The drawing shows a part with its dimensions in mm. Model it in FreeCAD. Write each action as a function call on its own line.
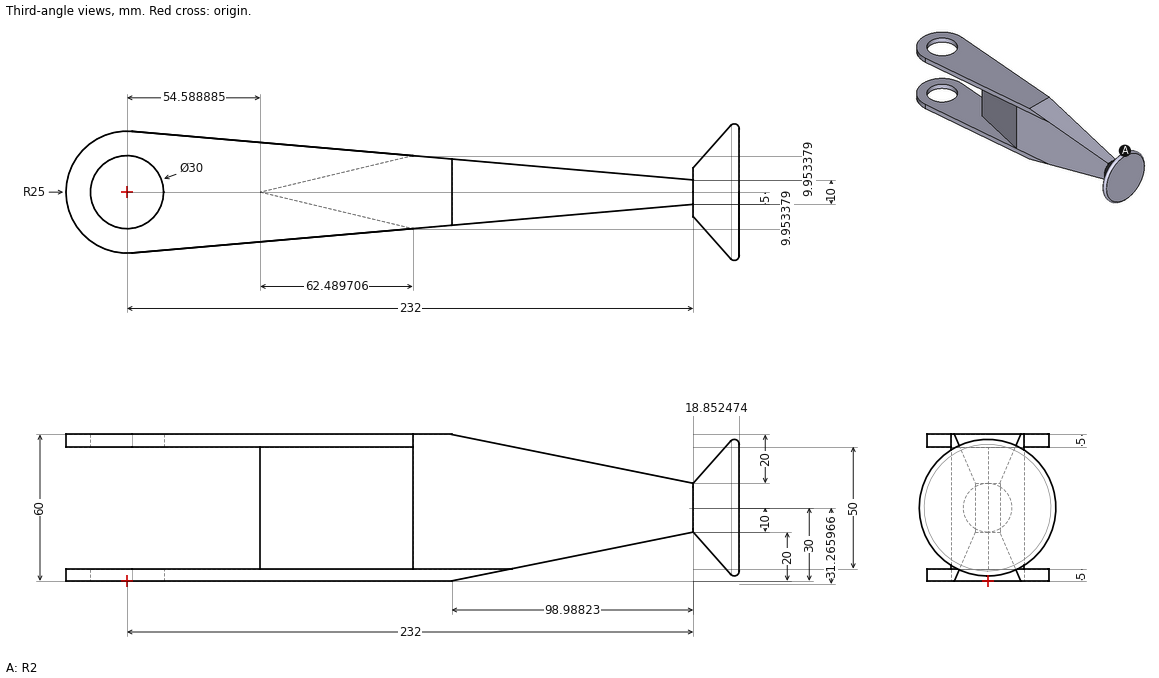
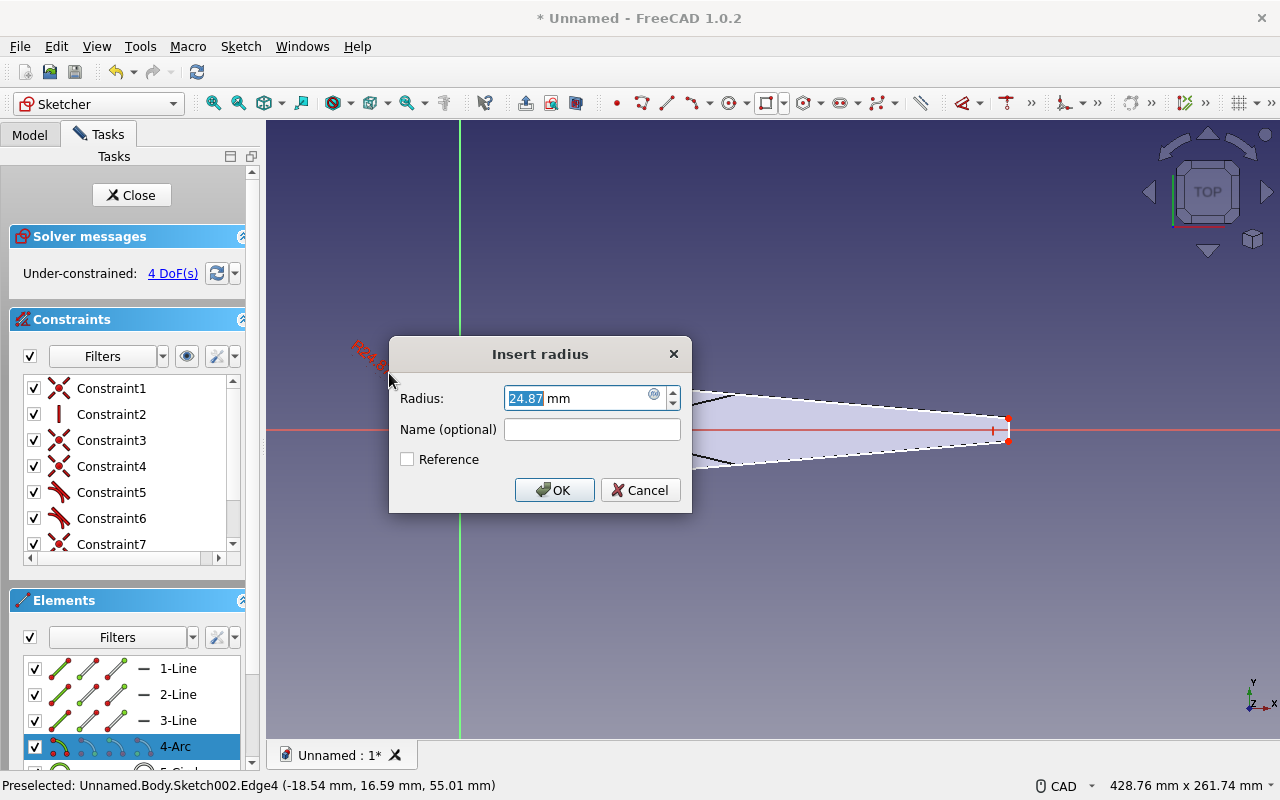
text(25)
key(Return)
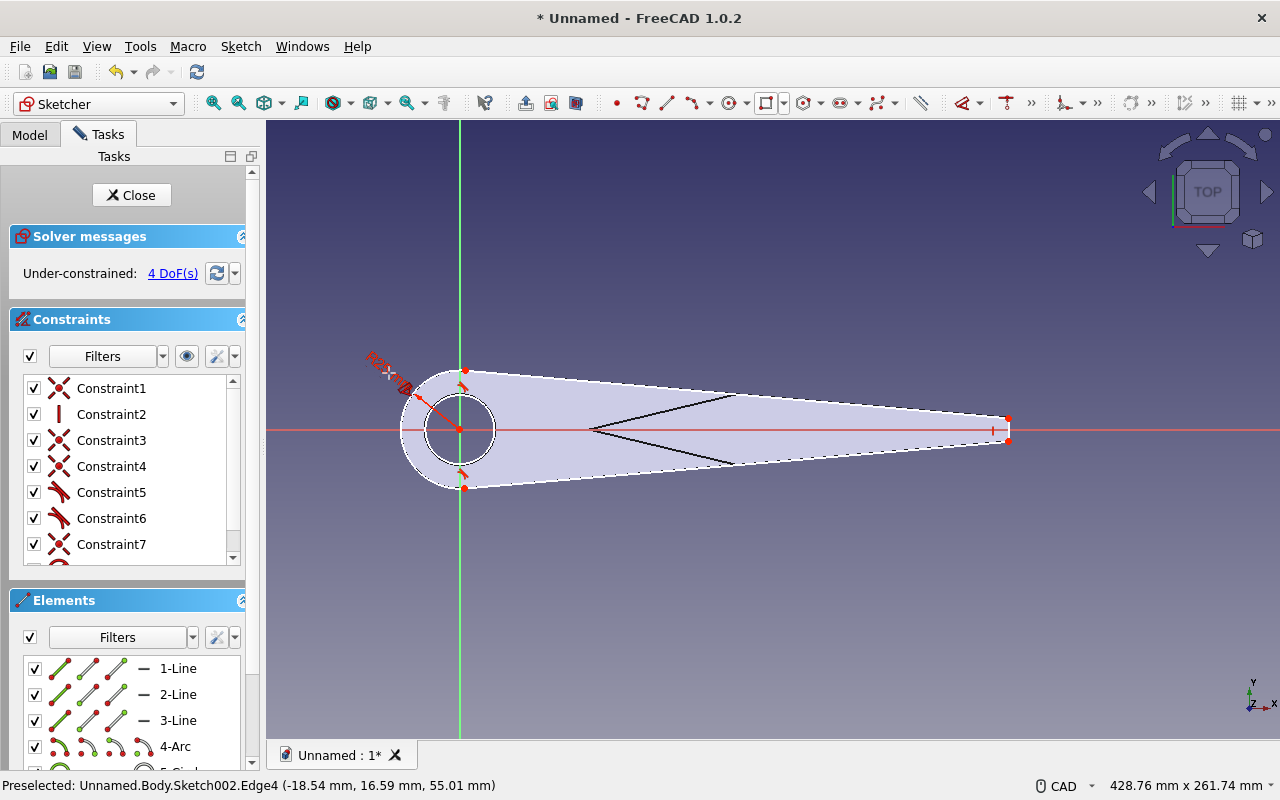
click(484, 405)
click(523, 410)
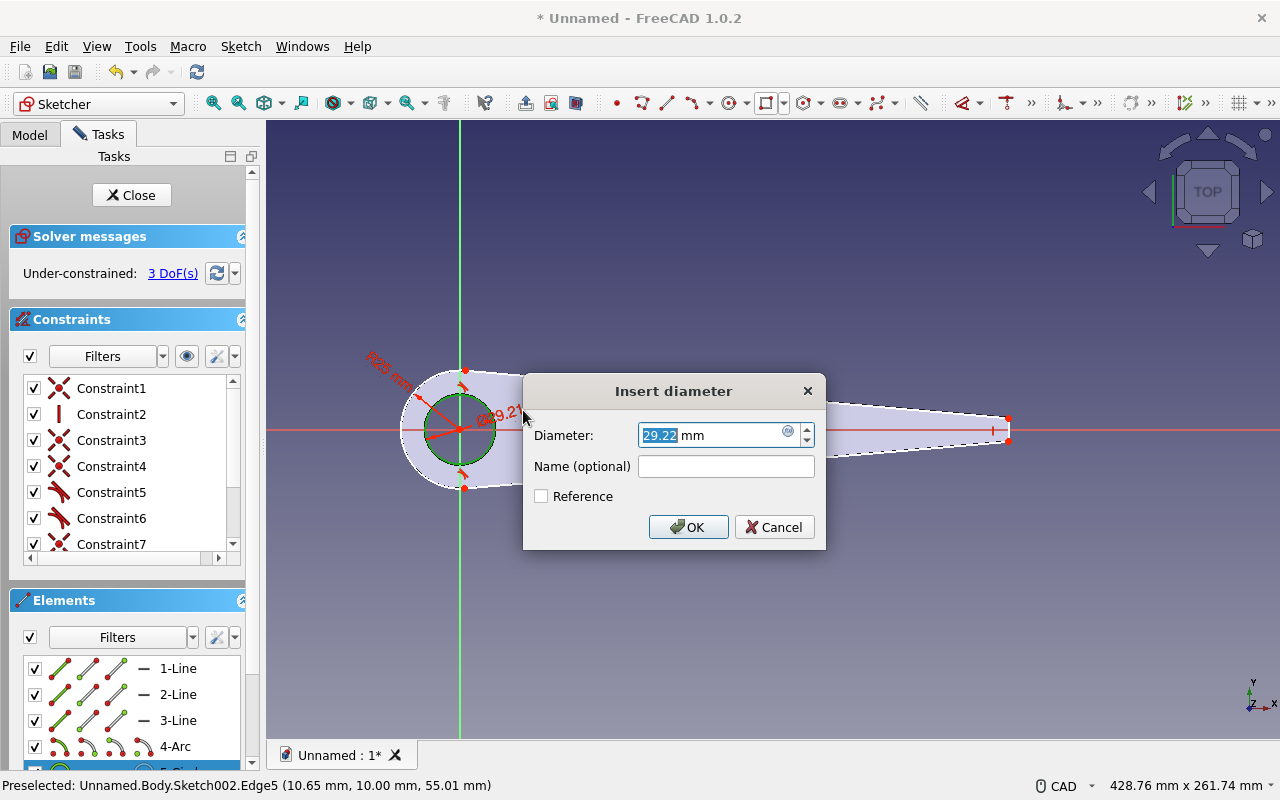
text(30)
key(Return)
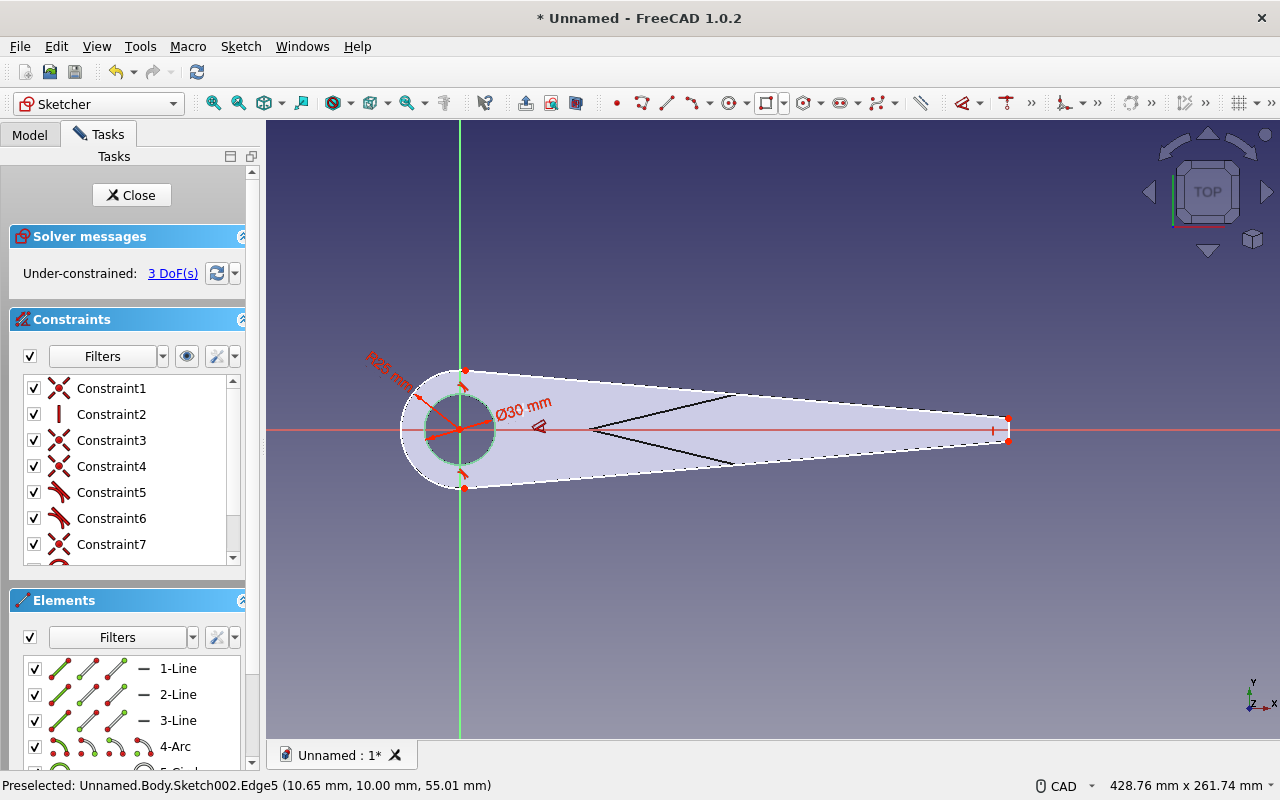
scroll(1009, 432, up, 3)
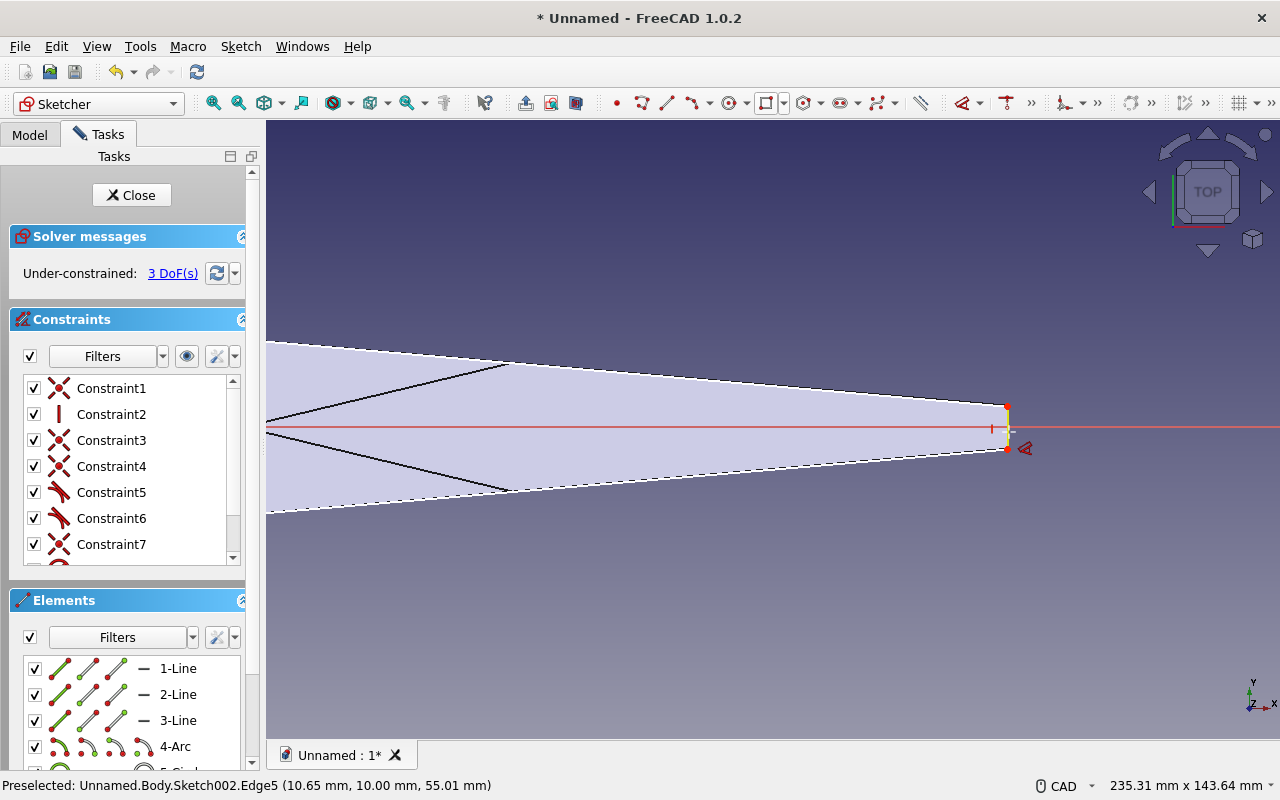
click(1008, 432)
click(1042, 413)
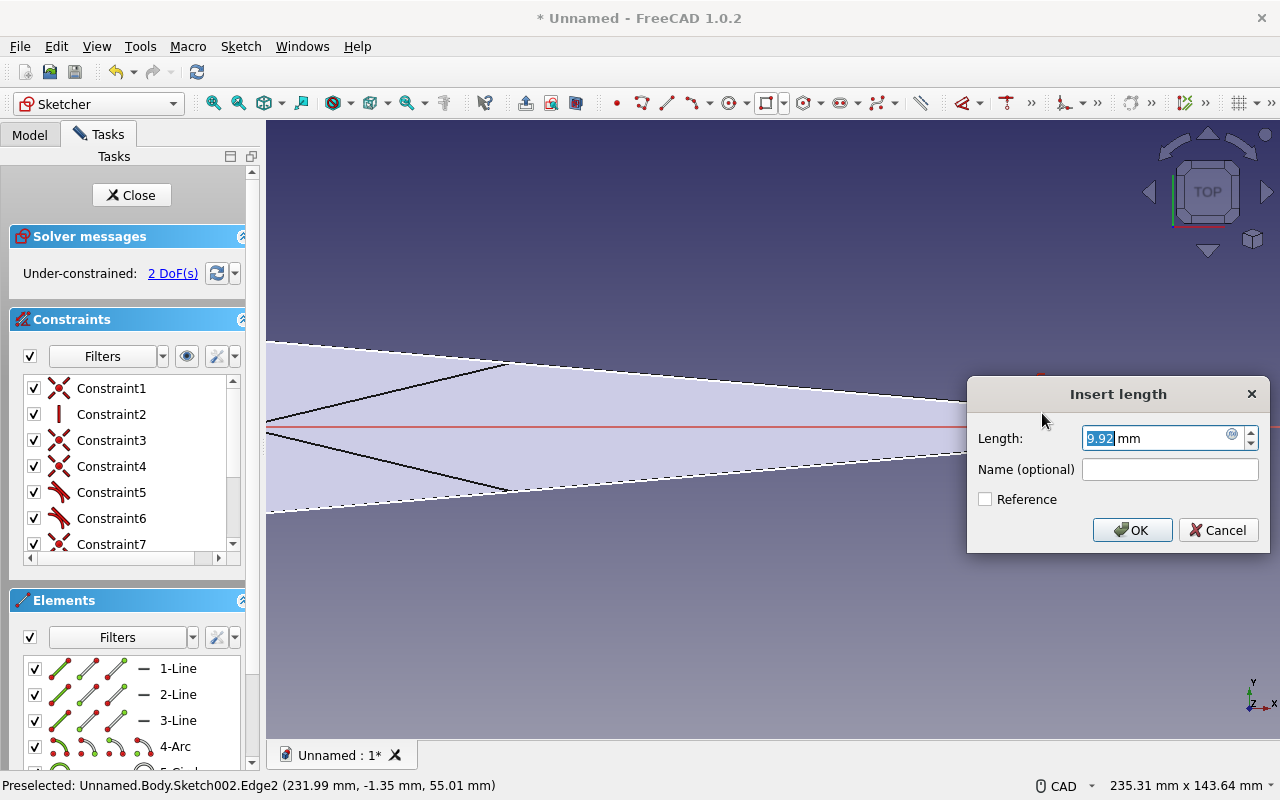
text(10)
key(Return)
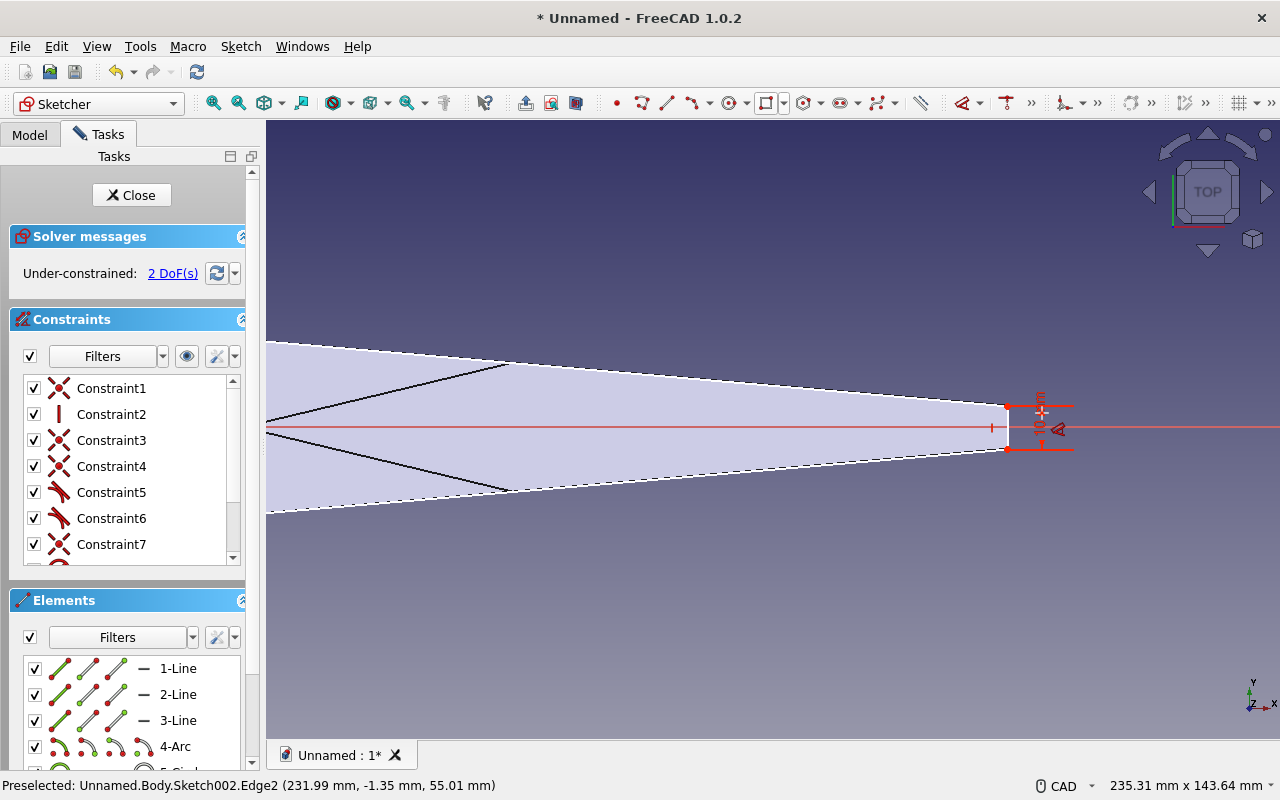
scroll(1008, 450, up, 4)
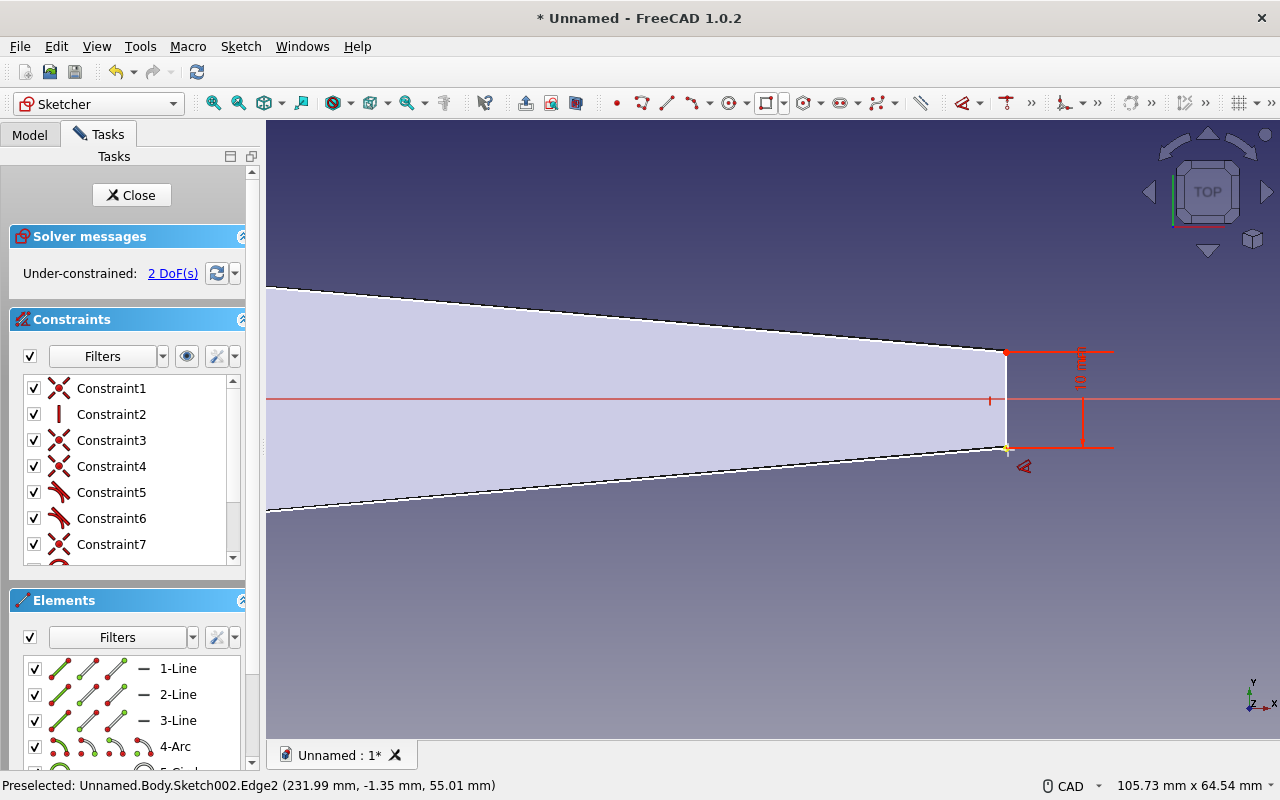
click(1006, 448)
click(1040, 423)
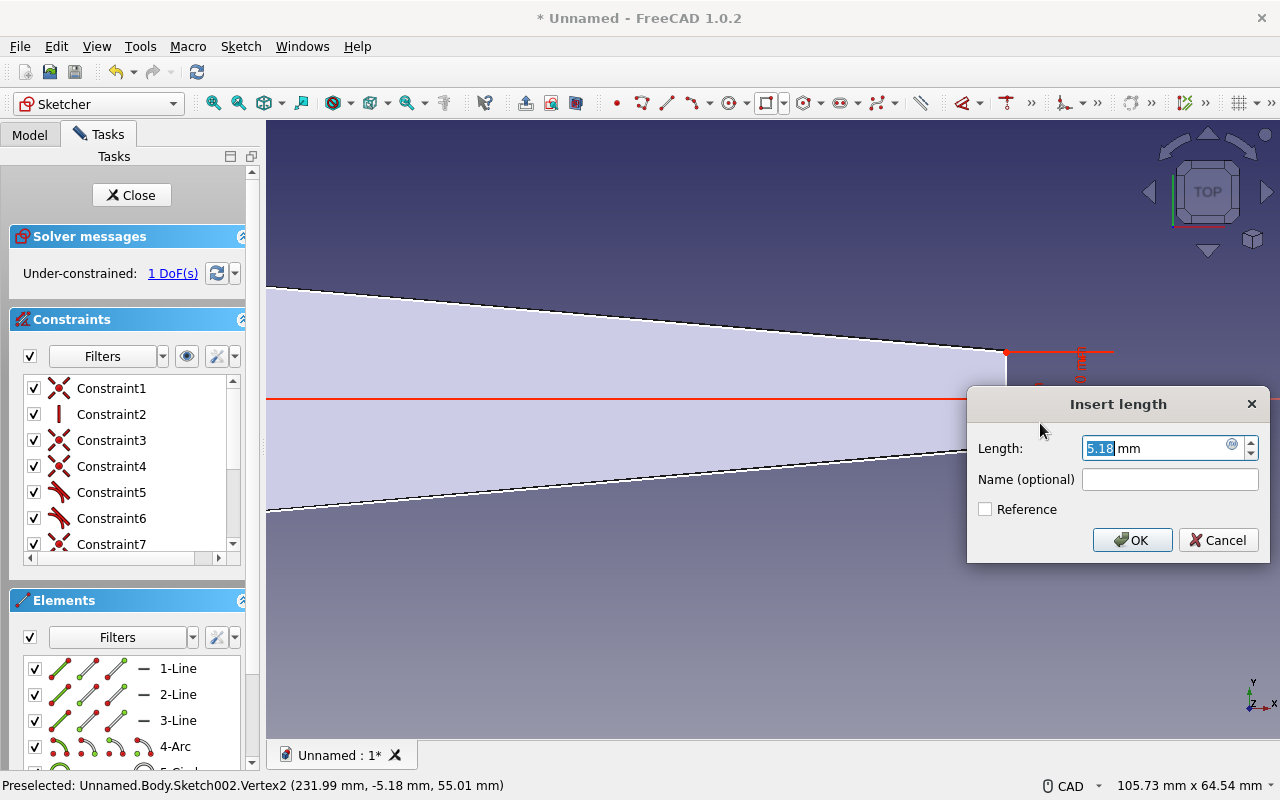
text(5)
key(Return)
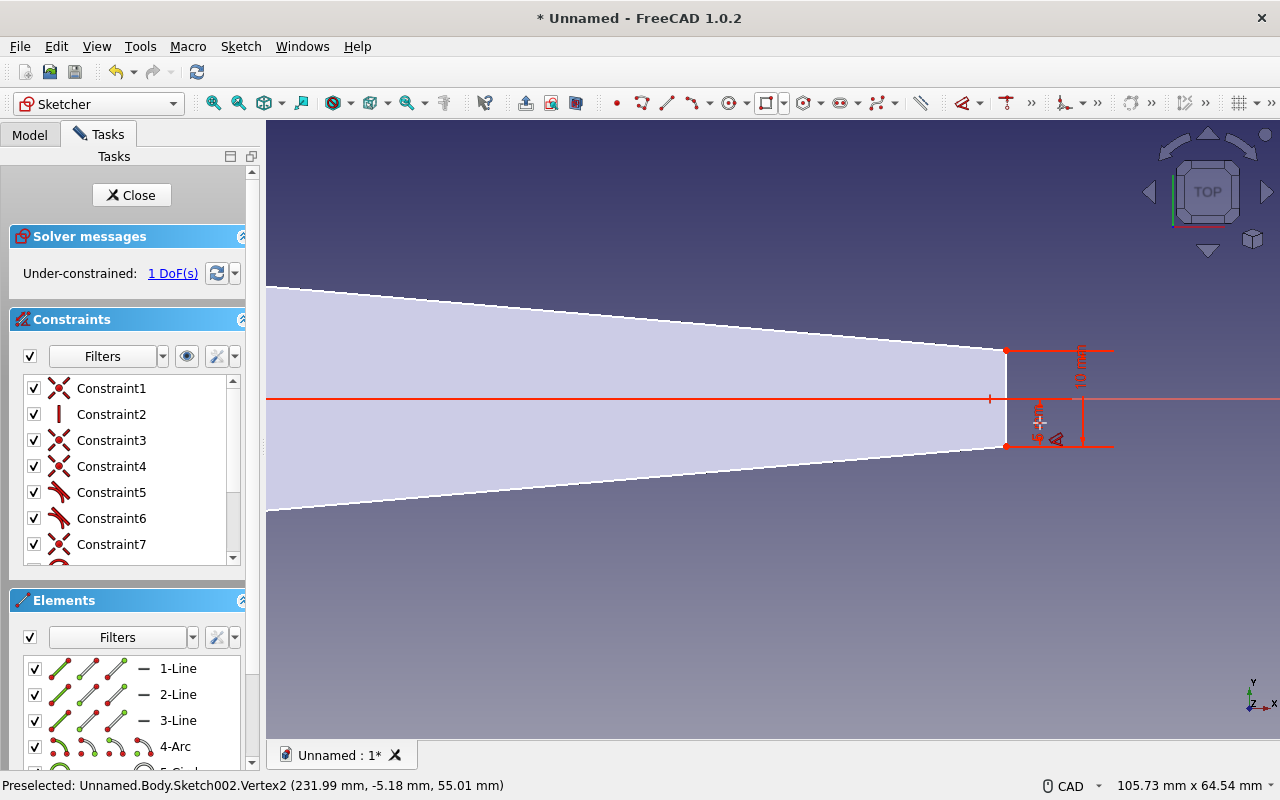
scroll(1009, 440, down, 7)